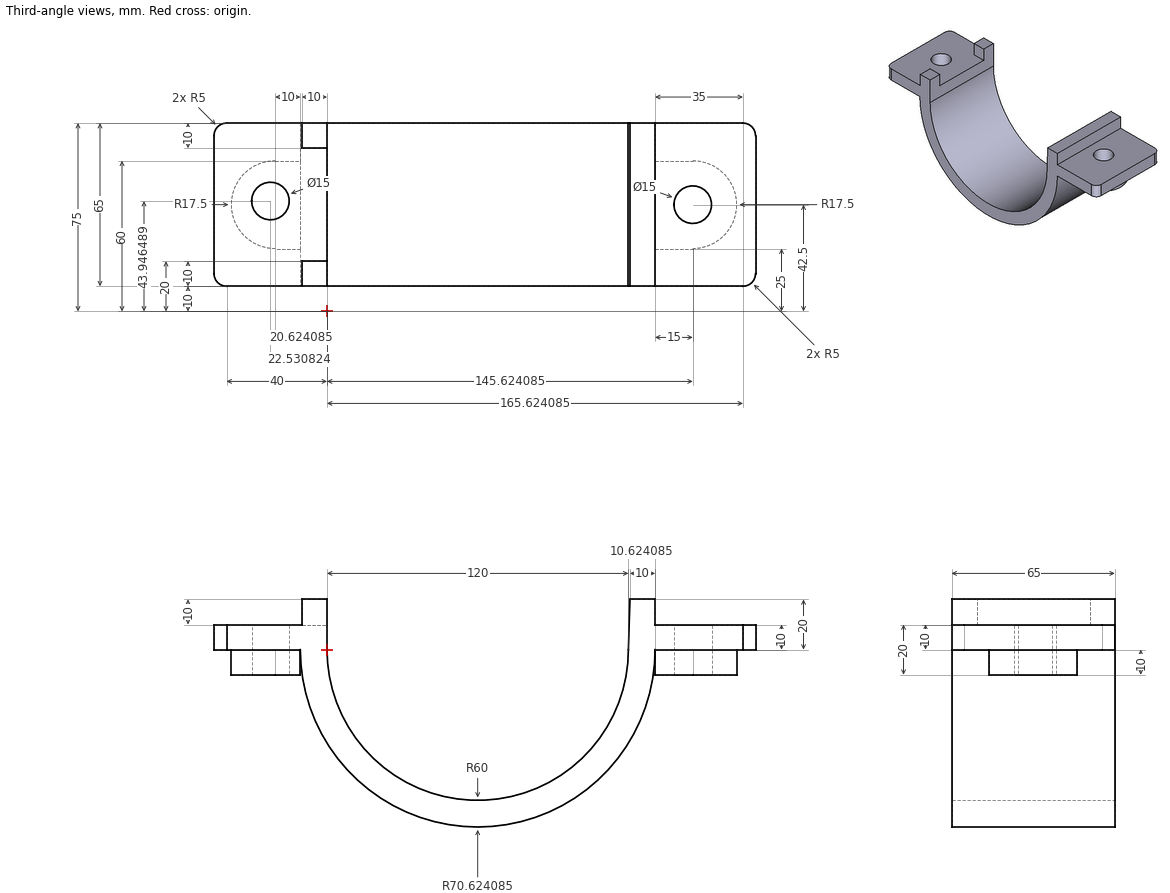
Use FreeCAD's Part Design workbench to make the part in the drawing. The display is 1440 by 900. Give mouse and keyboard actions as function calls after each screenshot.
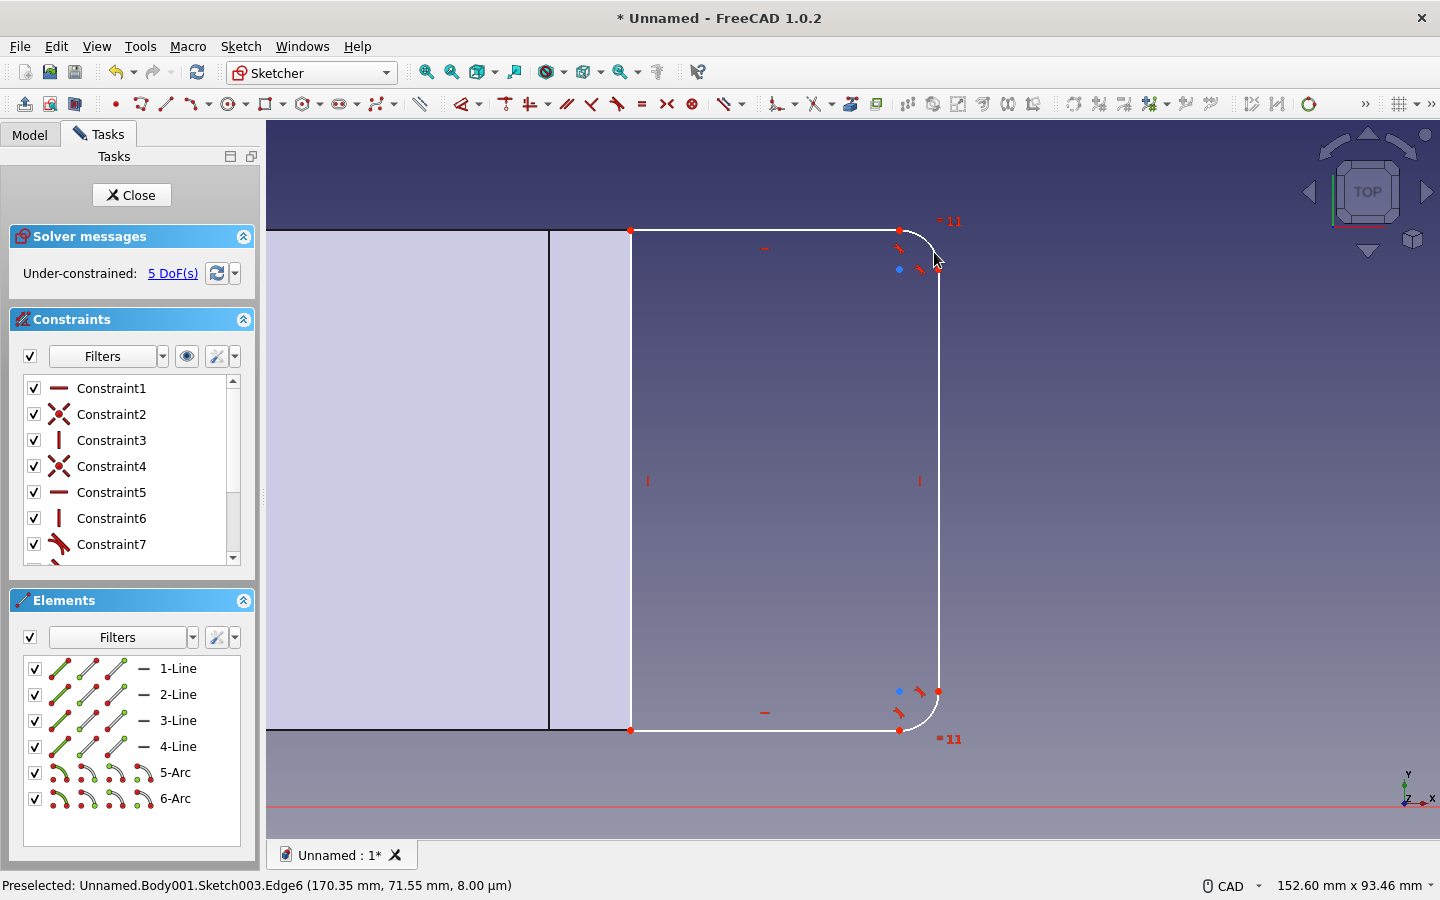
click(460, 104)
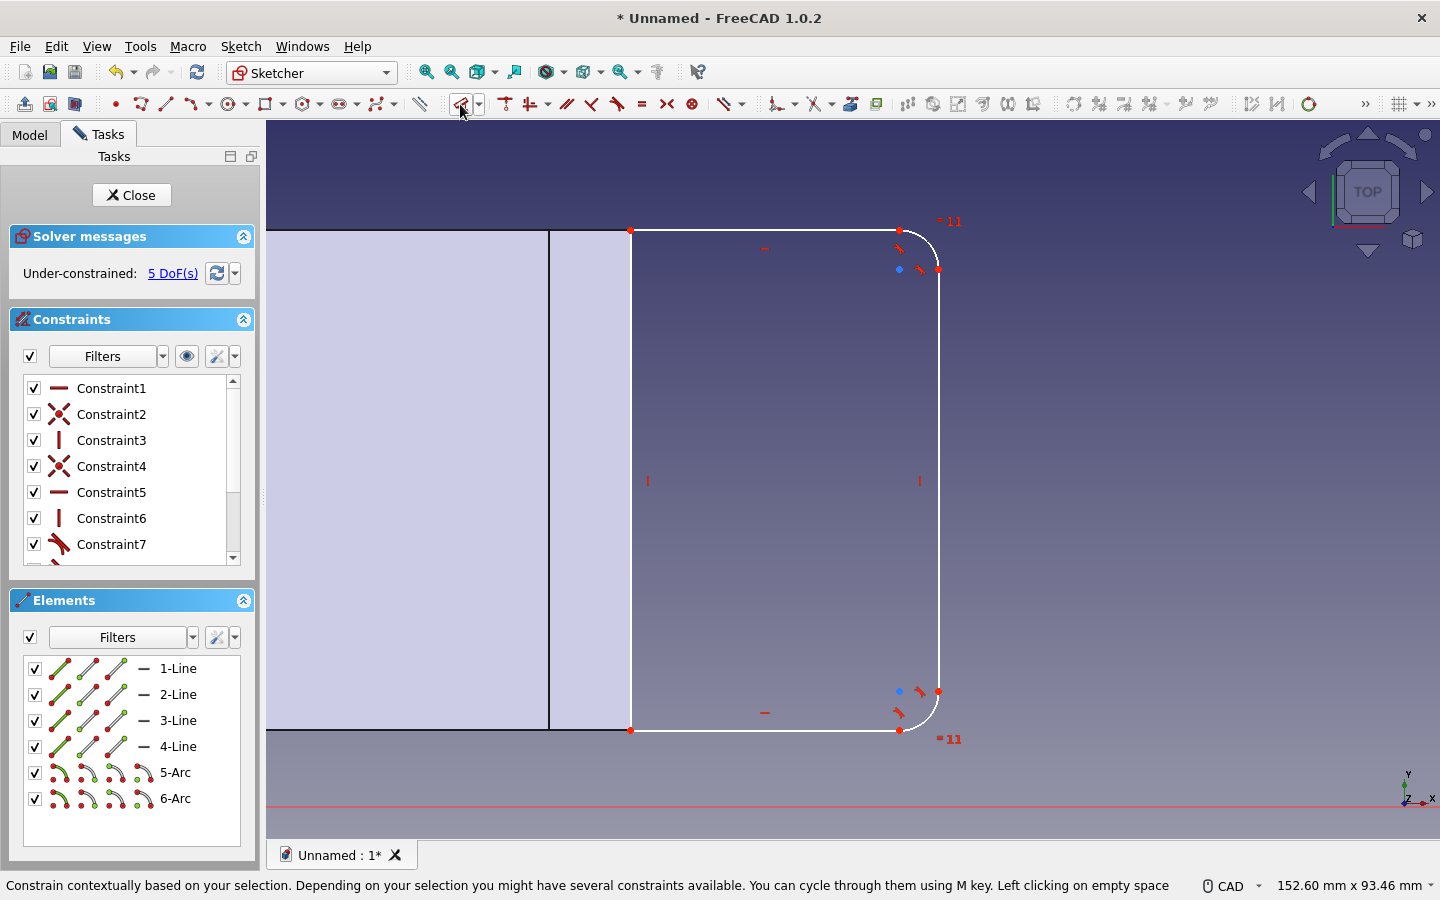
click(917, 727)
click(931, 756)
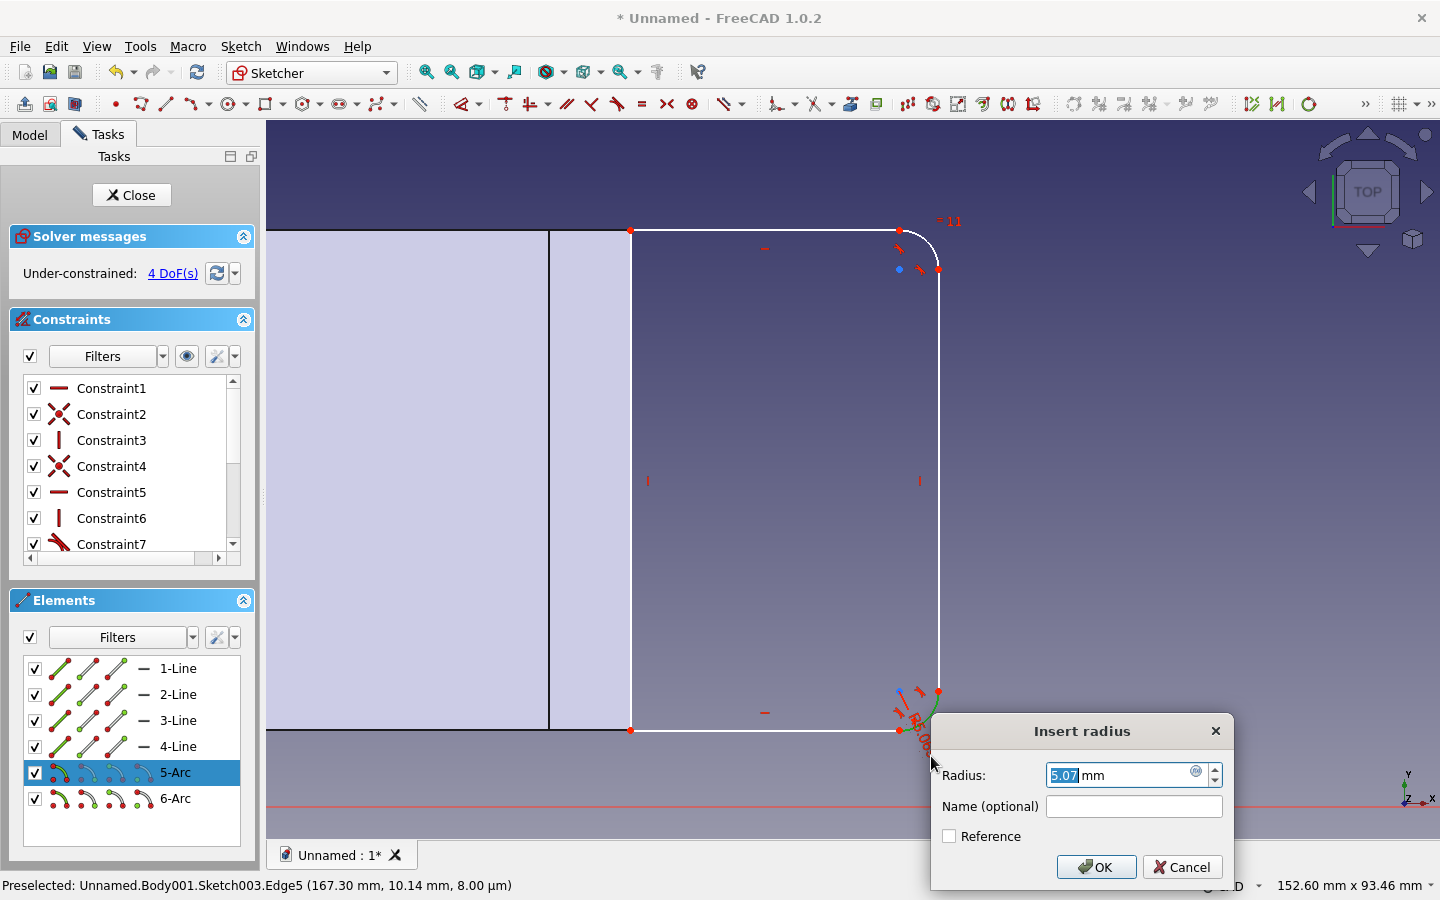
text(5)
key(Return)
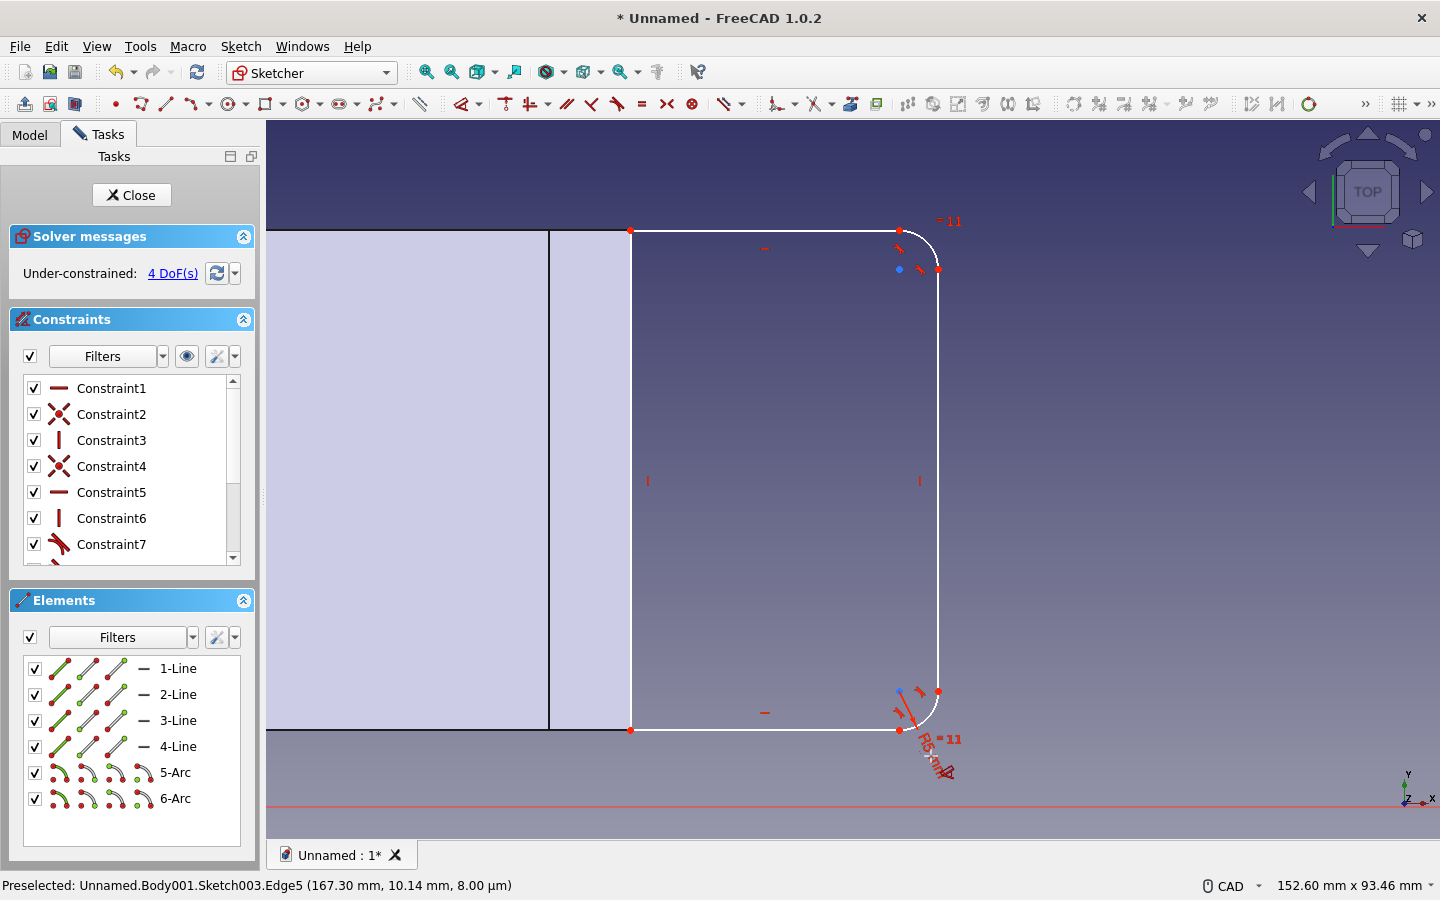
click(819, 231)
click(765, 197)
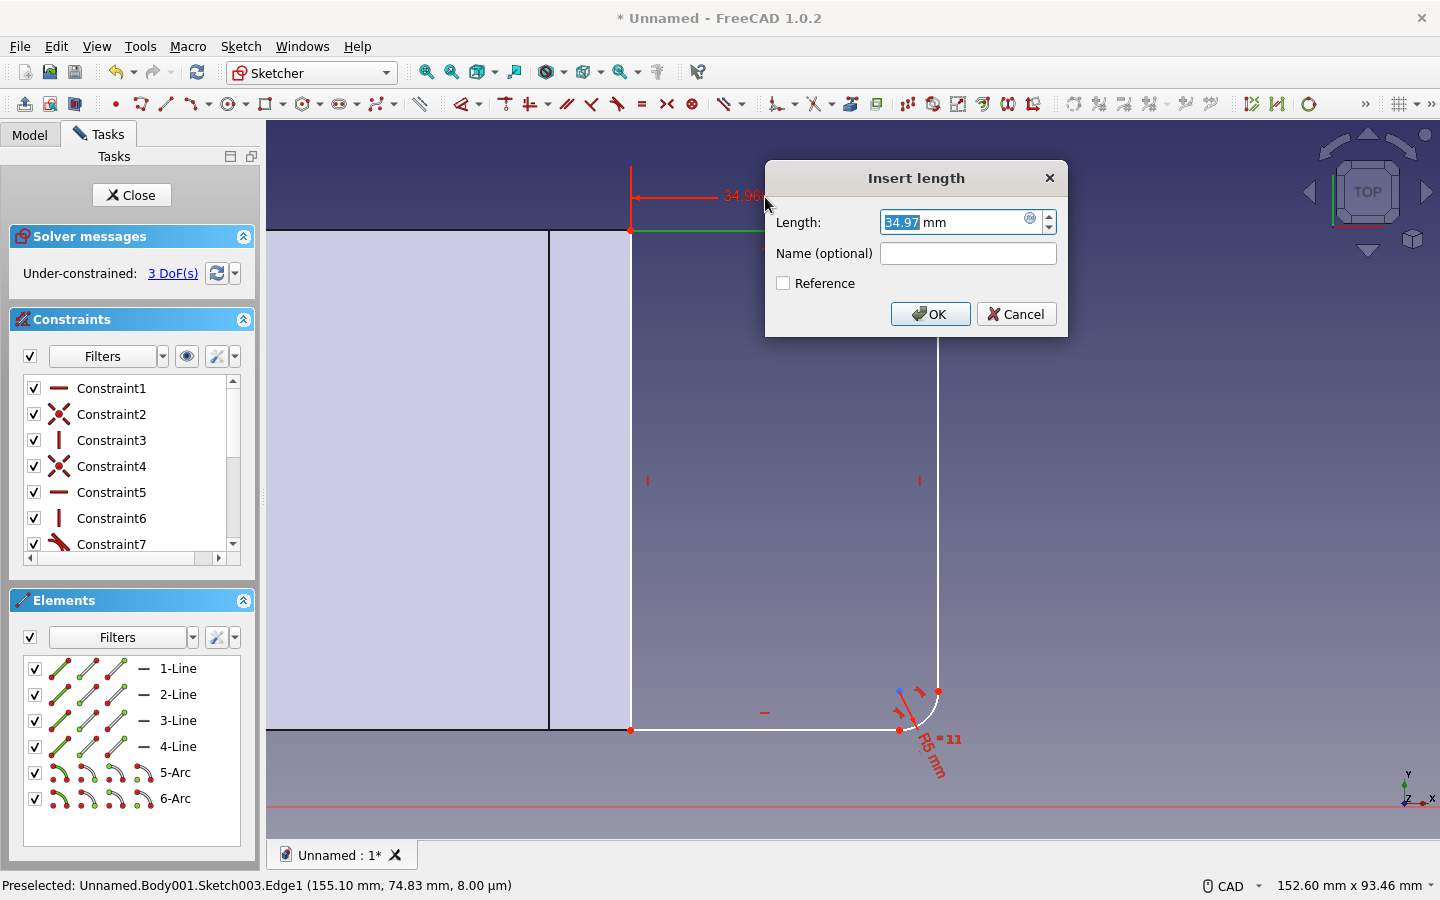
text(35)
key(Return)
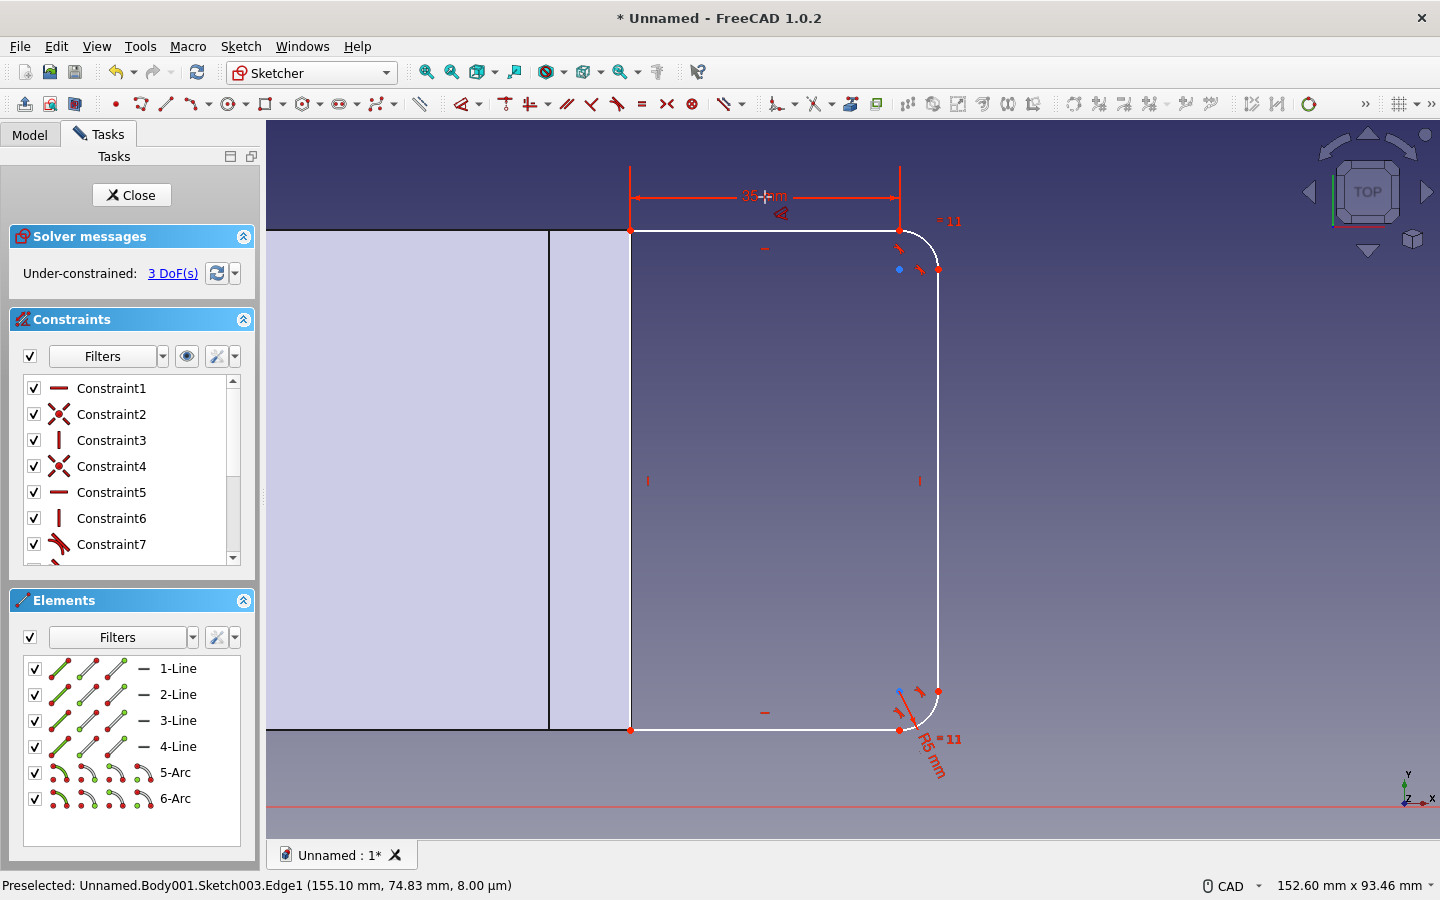
click(630, 381)
click(596, 481)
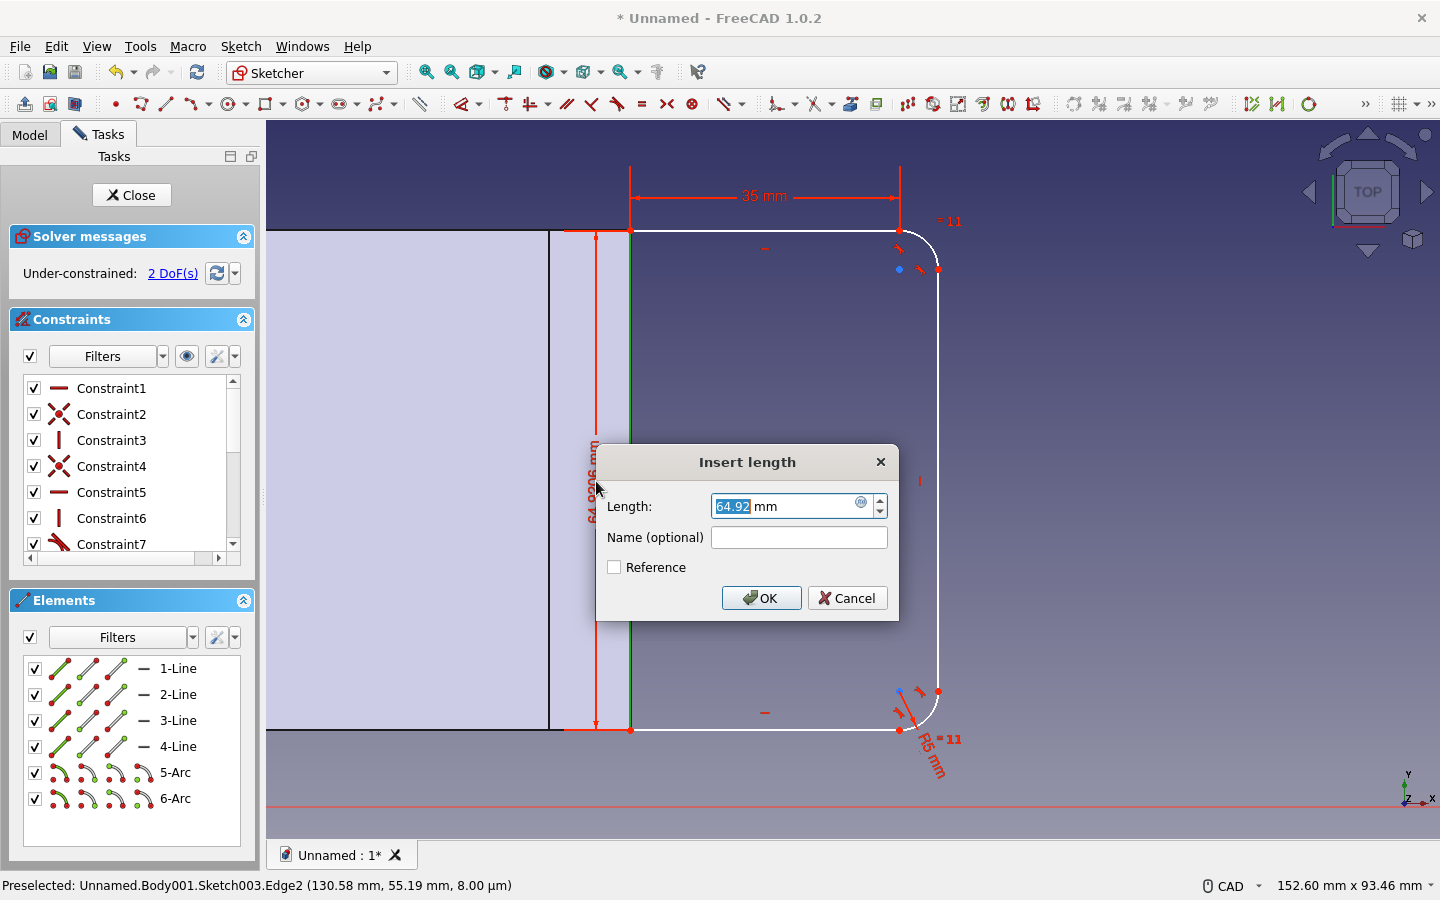
text(65)
key(Return)